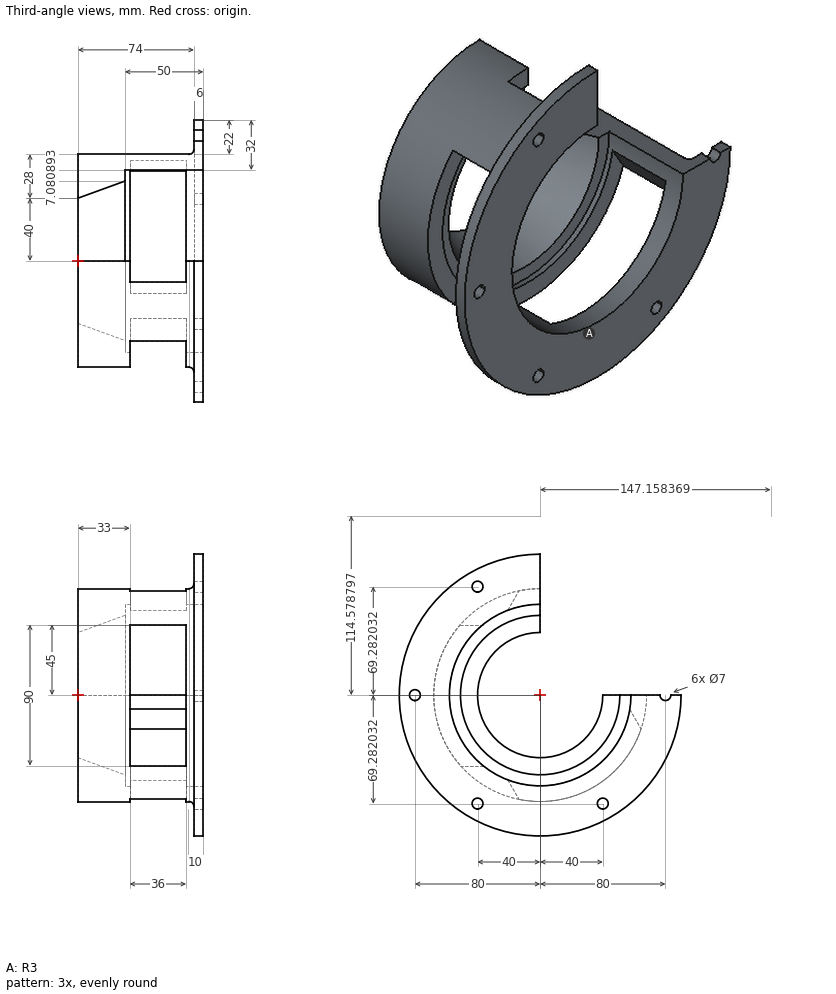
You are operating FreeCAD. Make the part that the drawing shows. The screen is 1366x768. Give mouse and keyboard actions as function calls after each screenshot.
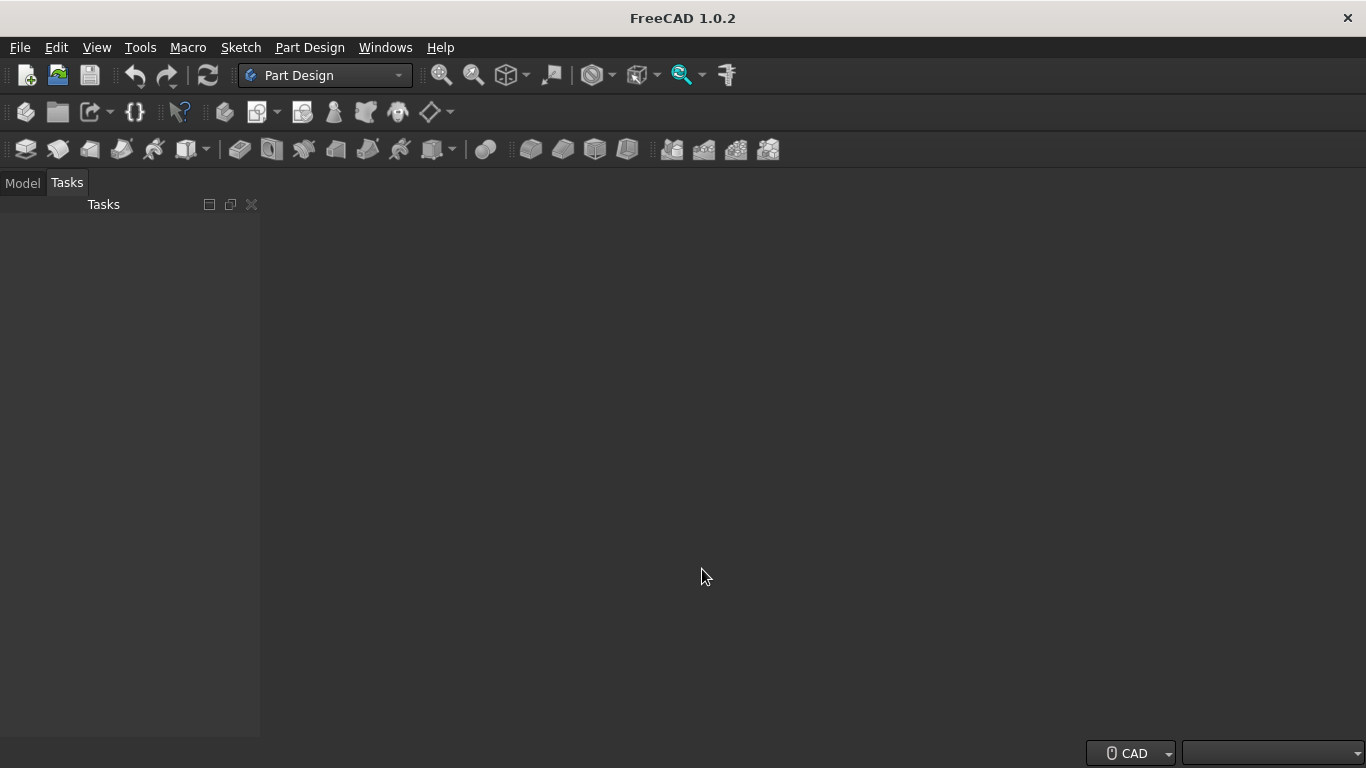
key(ctrl+n)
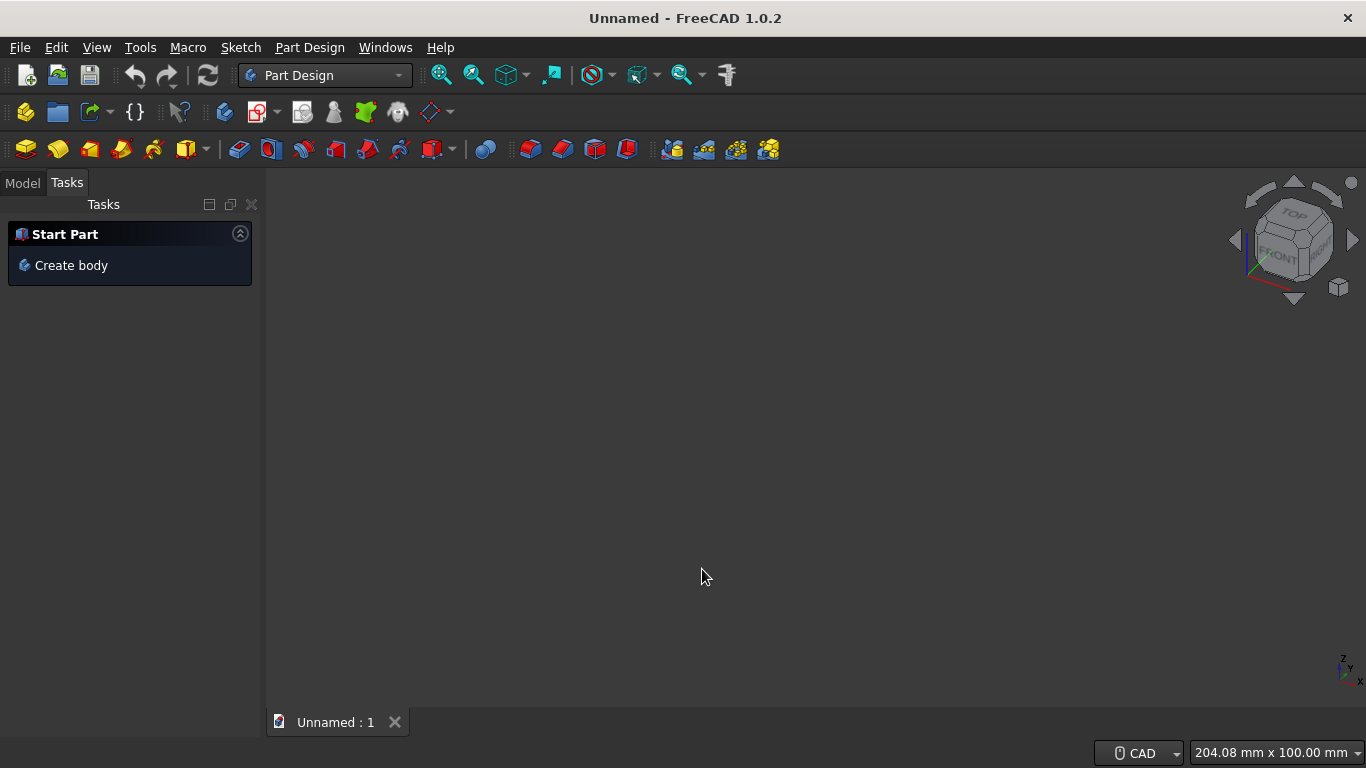
click(258, 112)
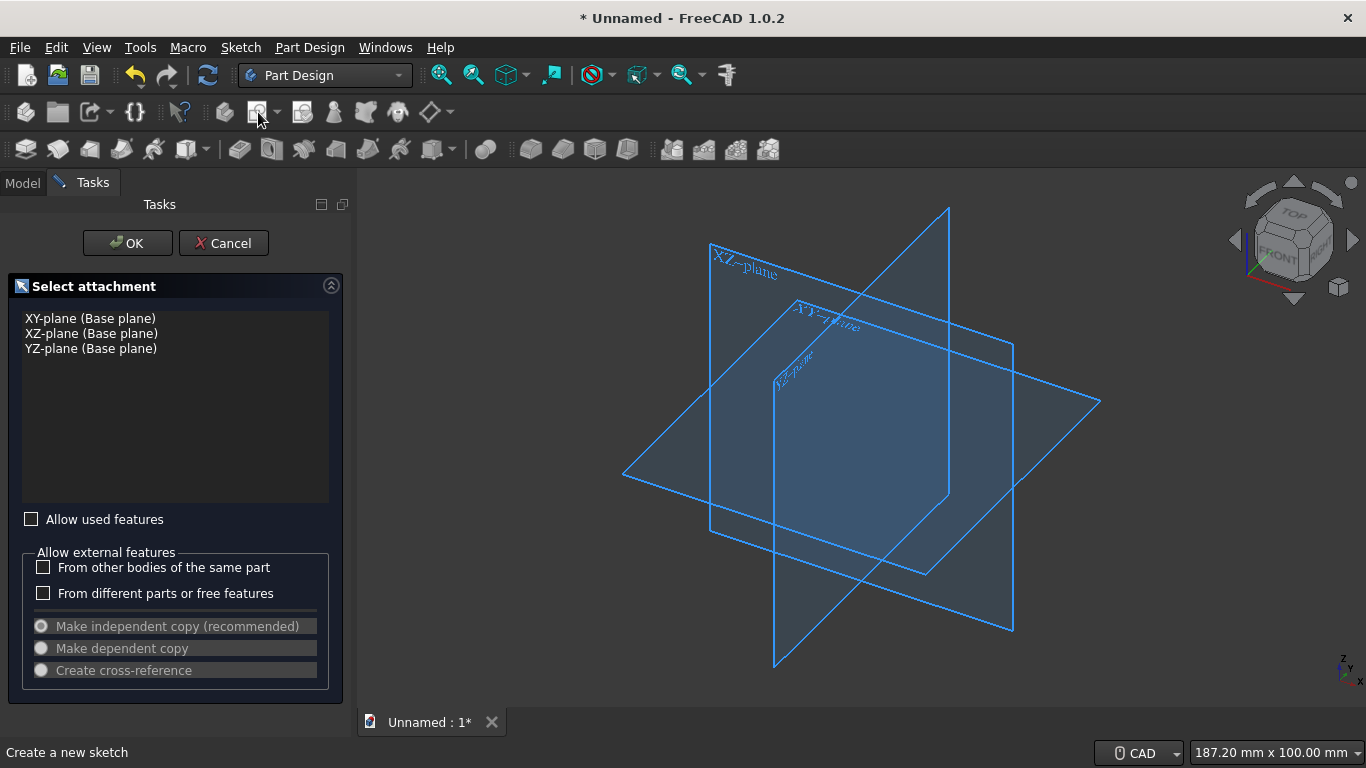
click(82, 318)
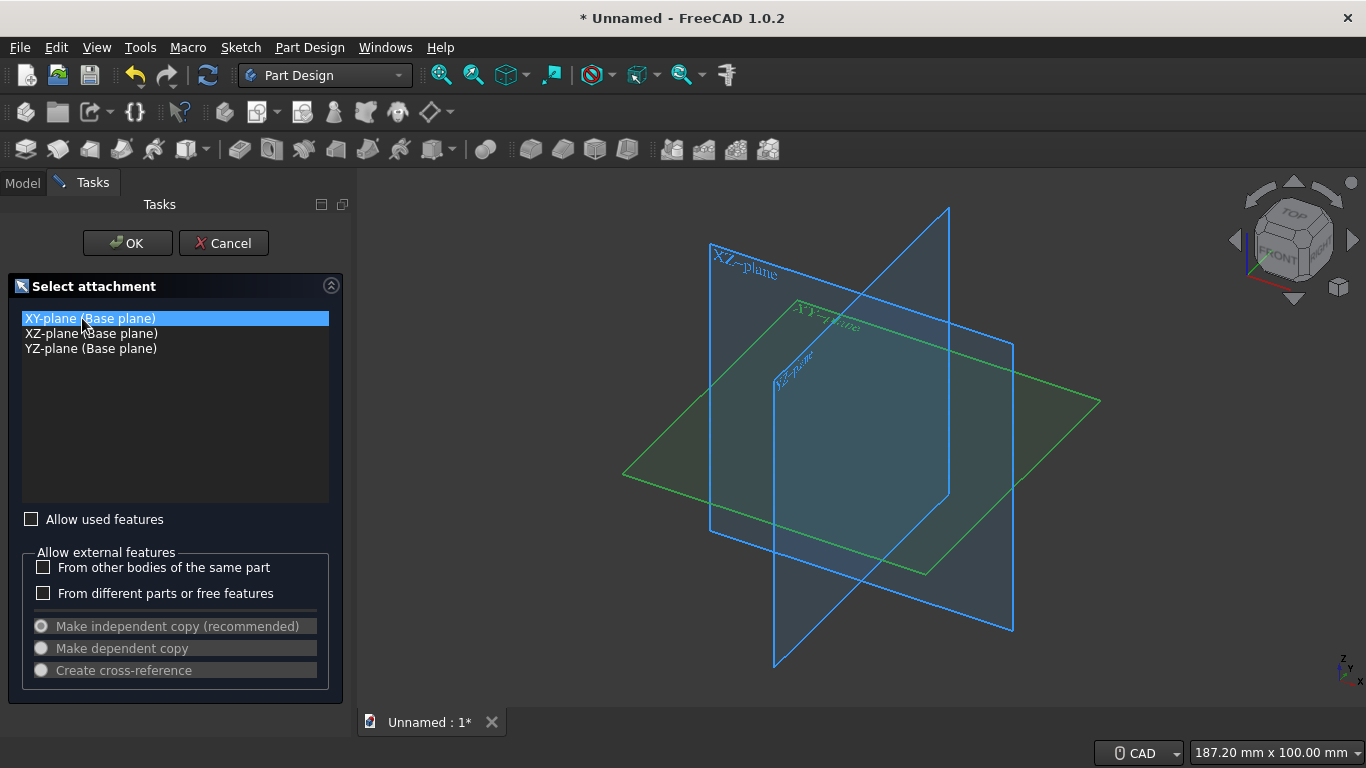
click(128, 243)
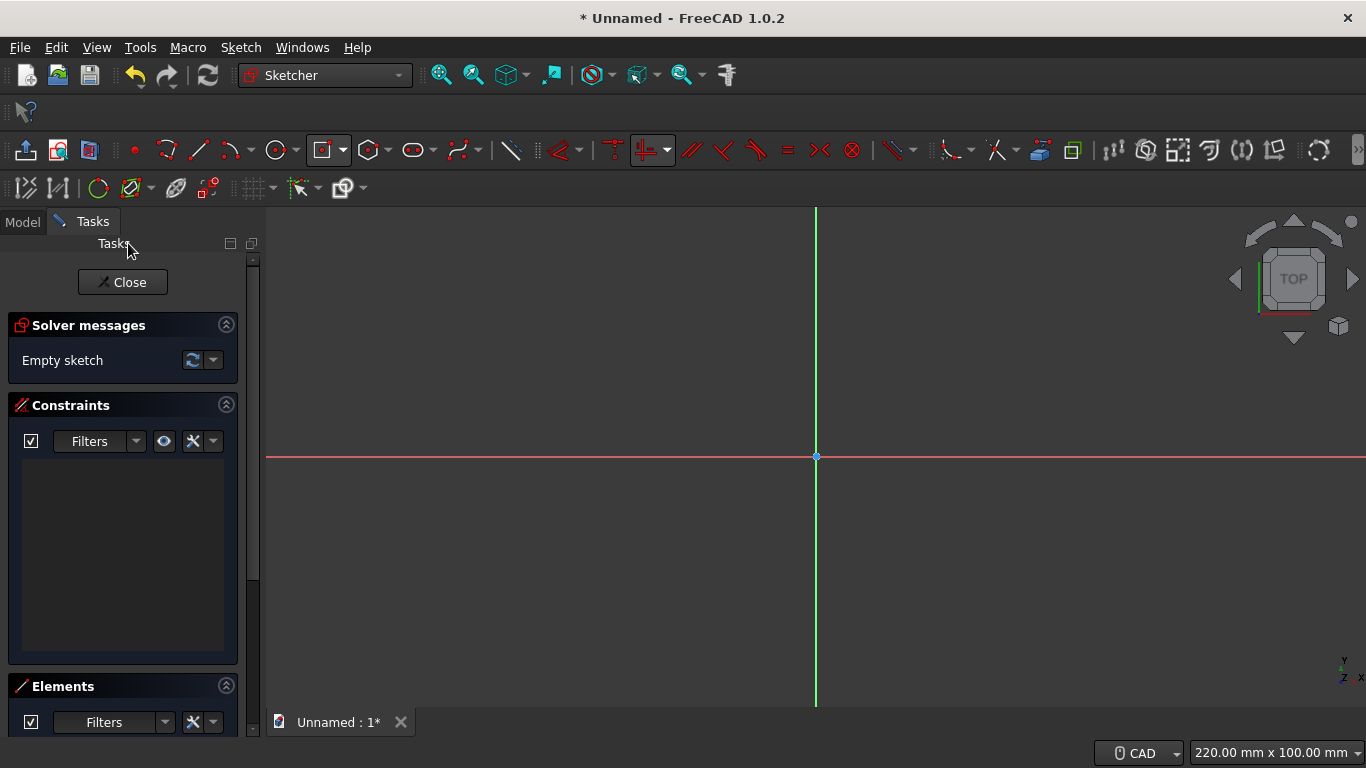
scroll(421, 679, down, 3)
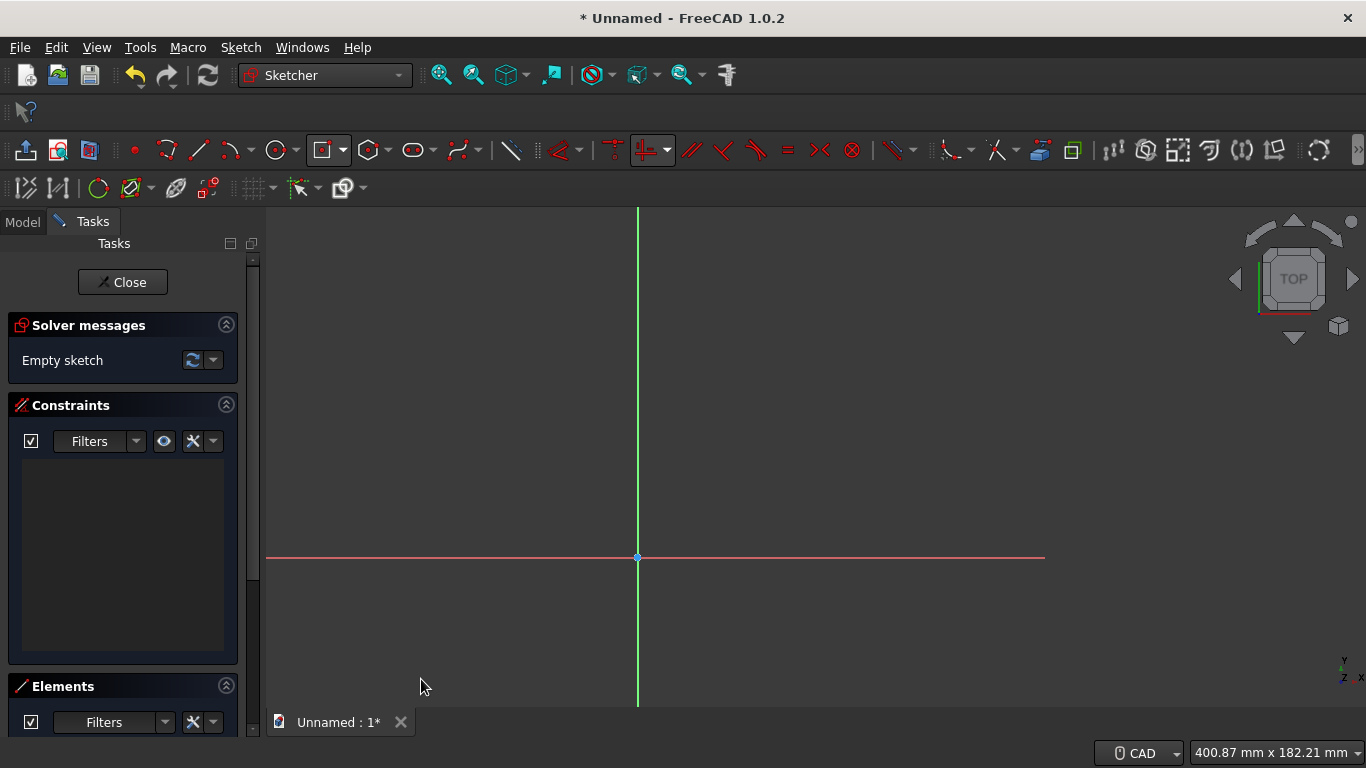
key(g)
key(m)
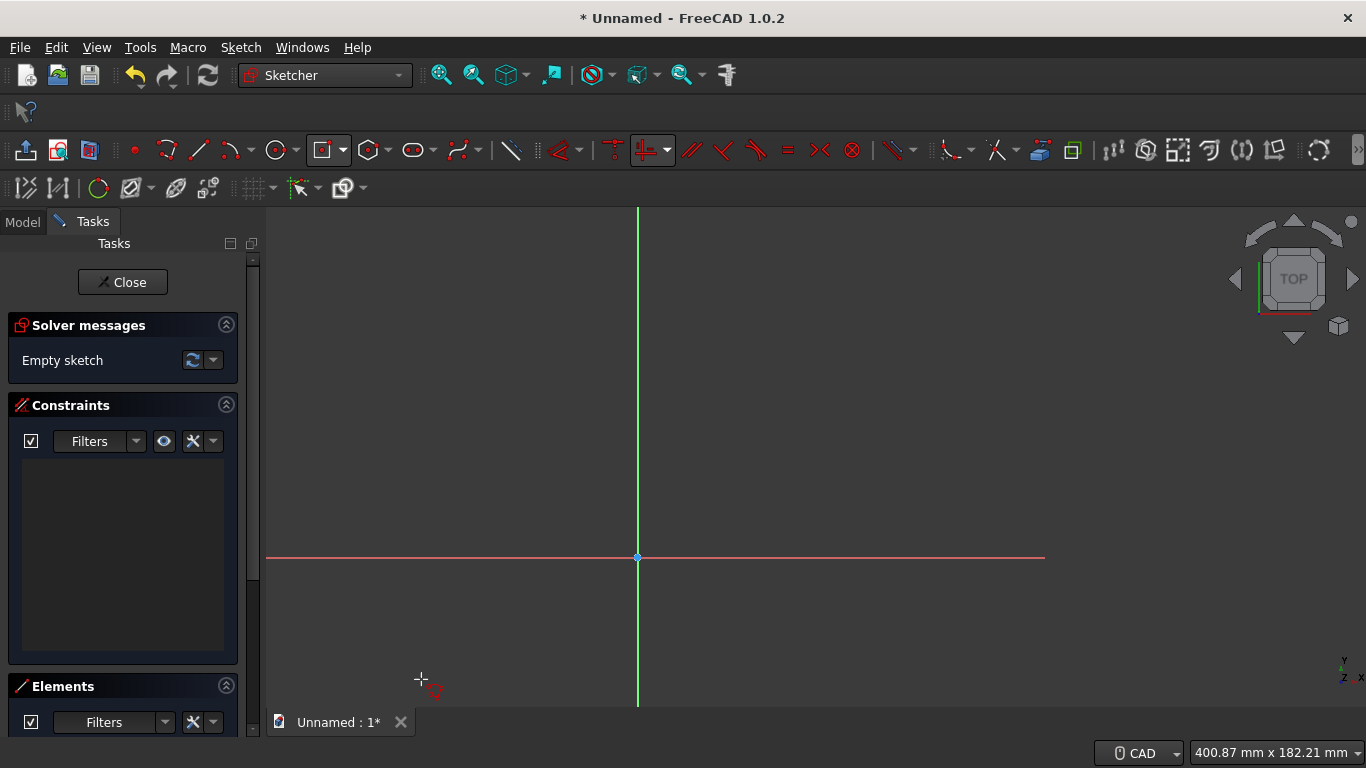
click(638, 448)
click(720, 418)
click(720, 398)
click(857, 398)
click(857, 311)
click(841, 311)
click(841, 371)
click(647, 371)
click(638, 449)
key(Escape)
key(Escape)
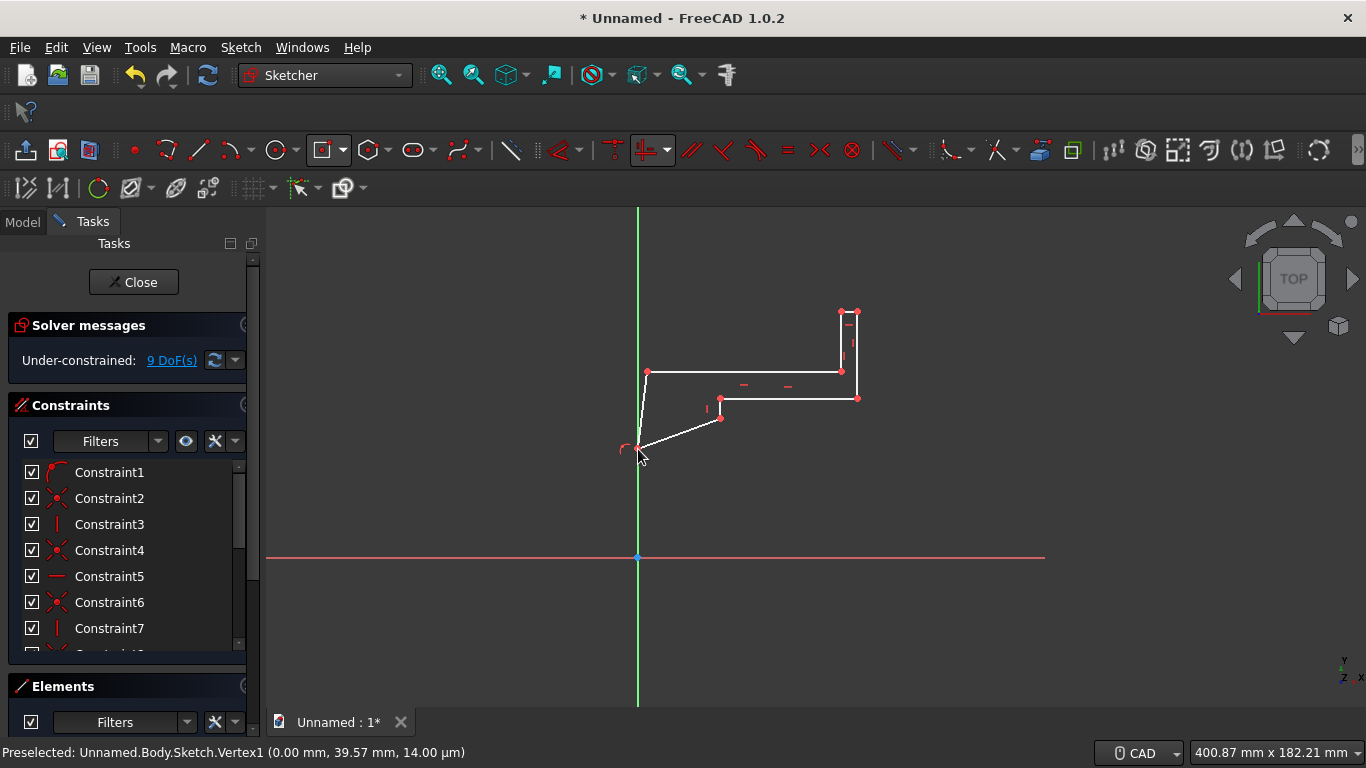
click(641, 426)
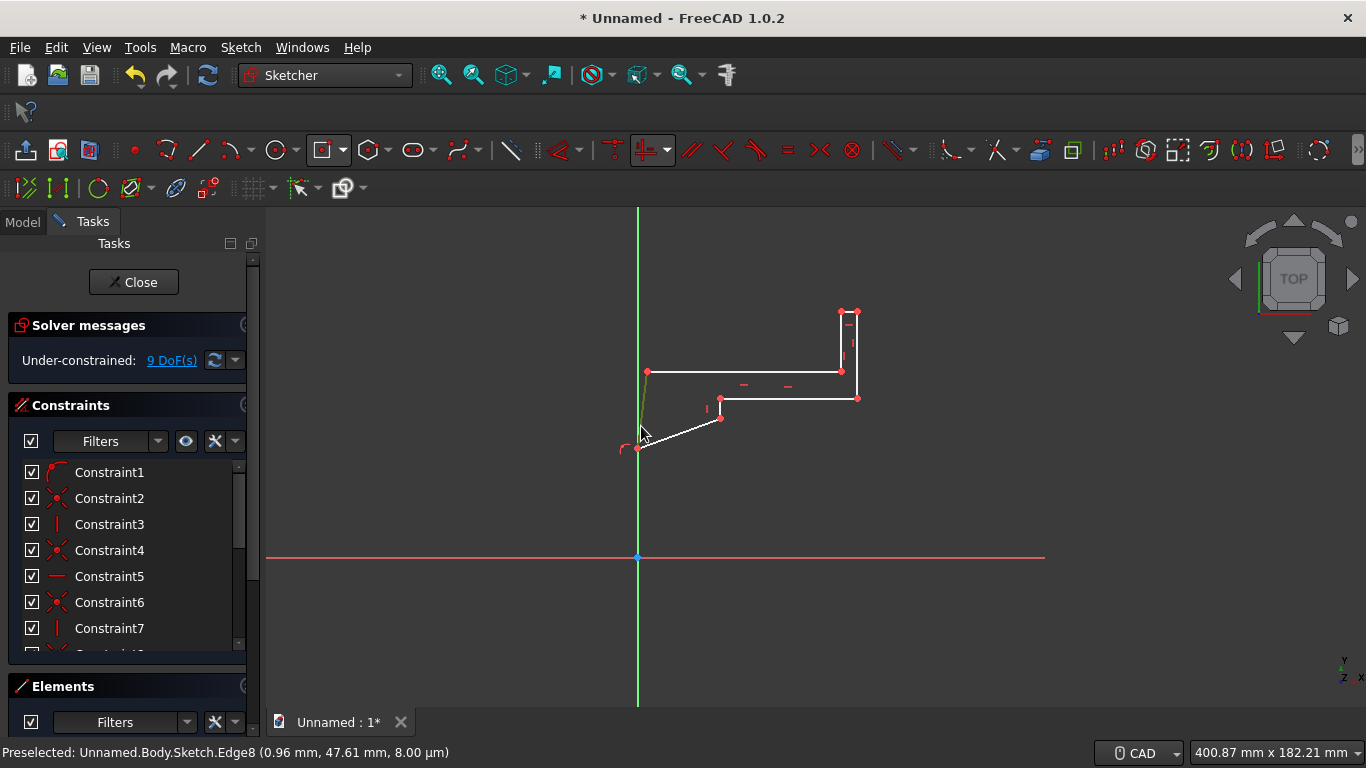
key(v)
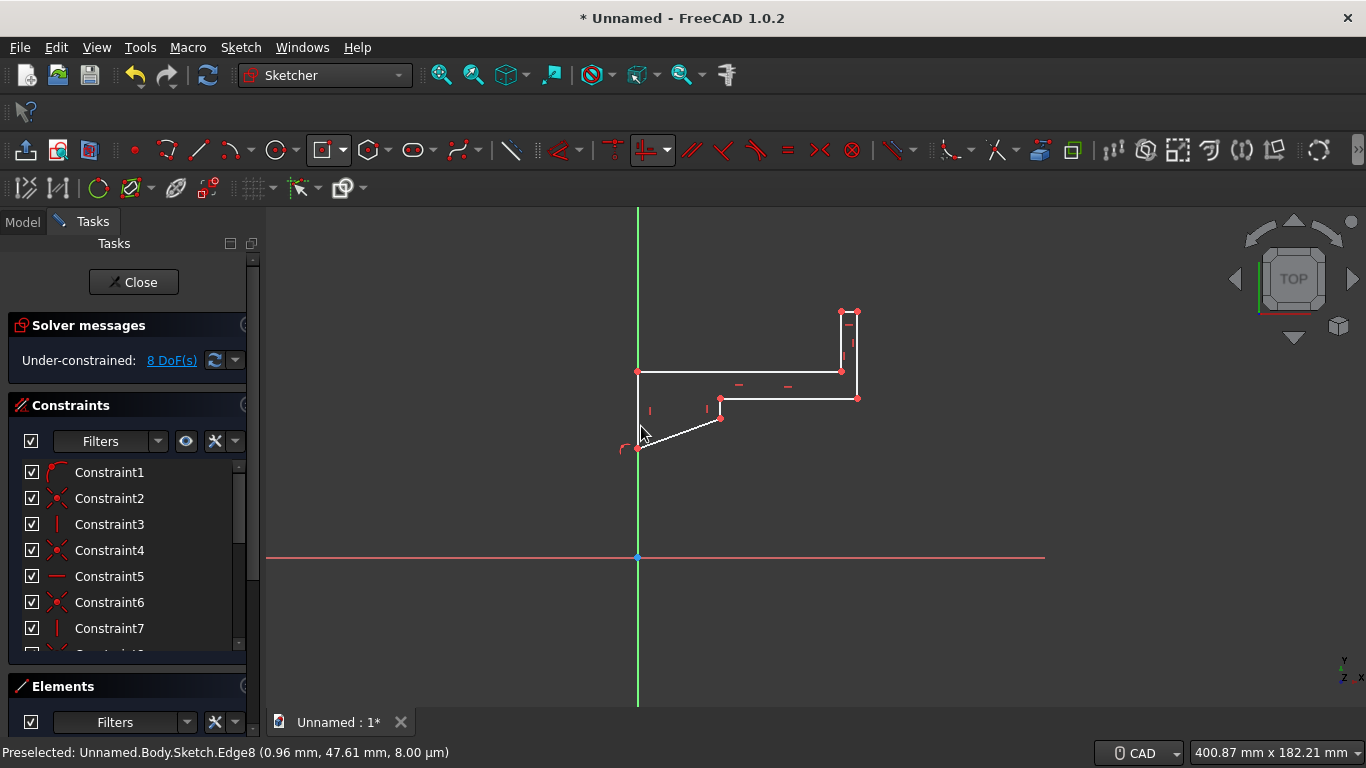
scroll(849, 312, up, 5)